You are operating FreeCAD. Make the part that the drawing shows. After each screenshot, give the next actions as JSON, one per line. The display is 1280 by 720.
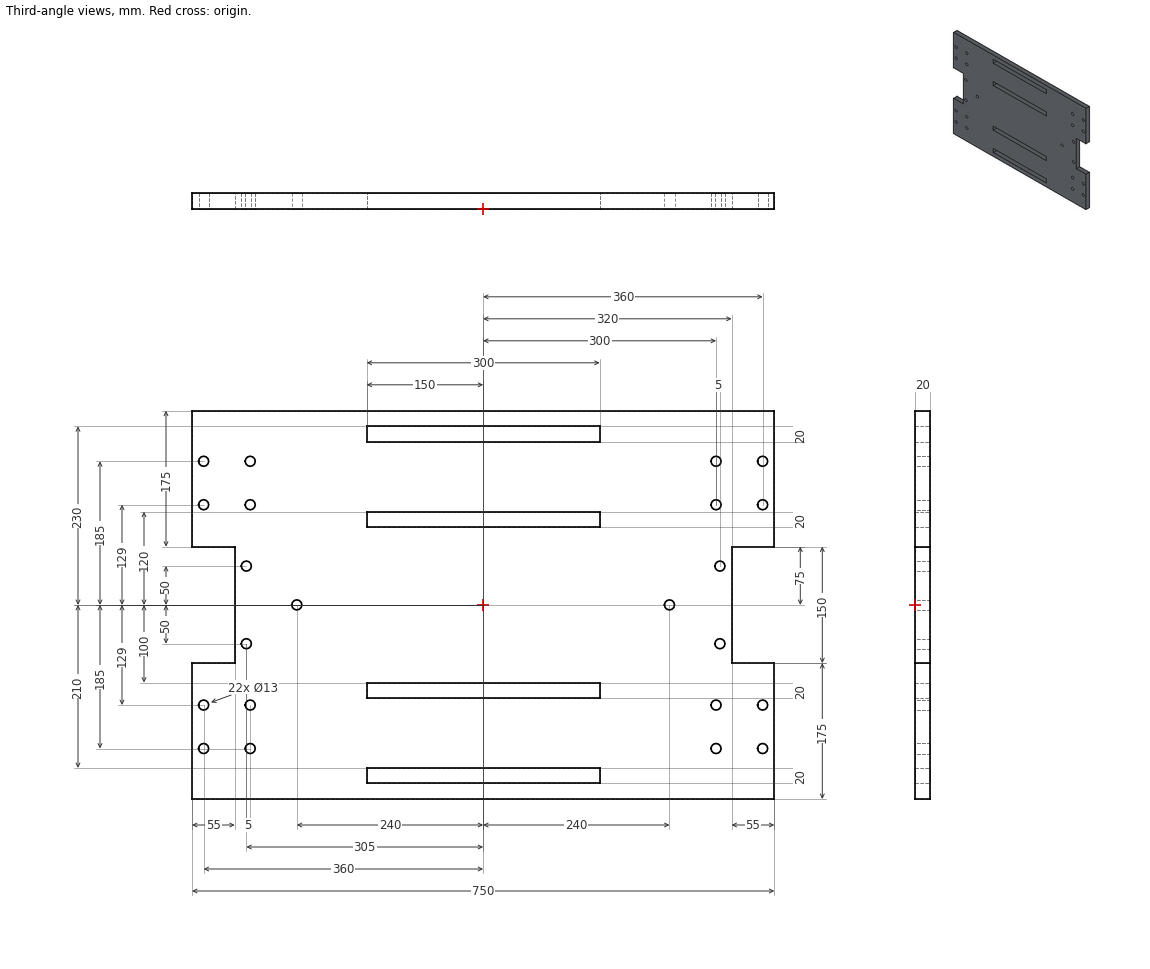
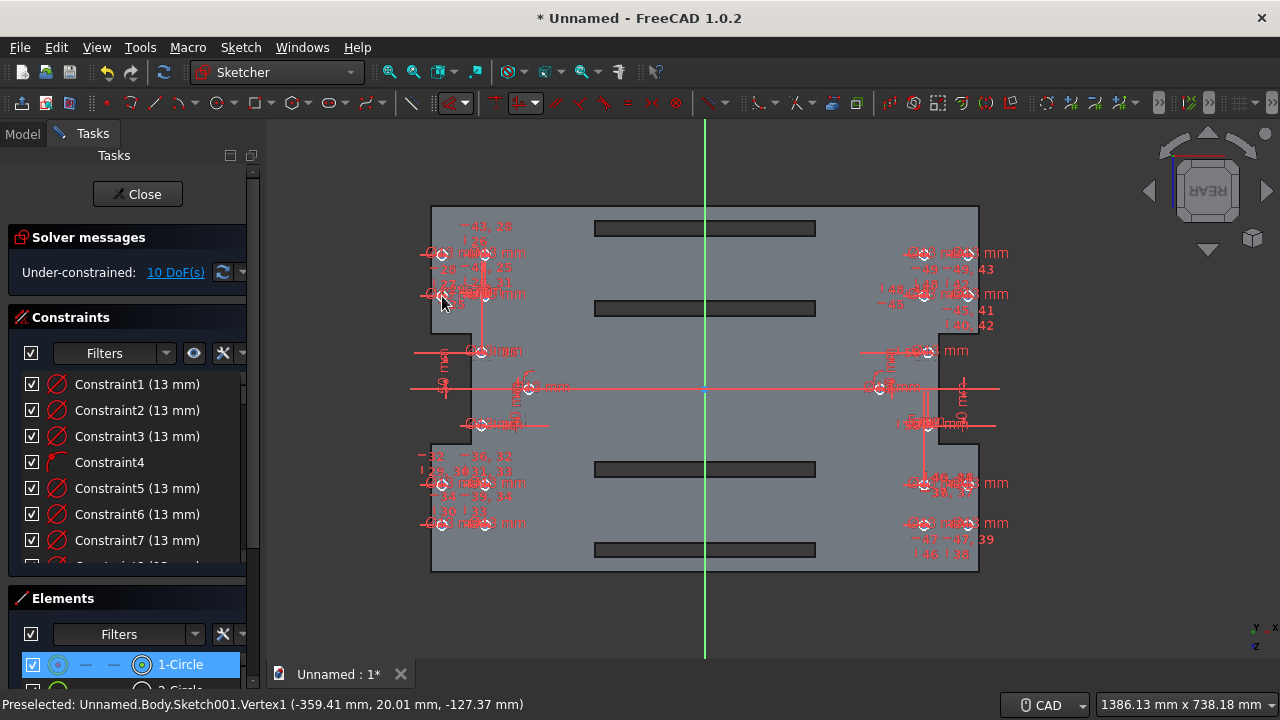
{"action": "key", "text": "l"}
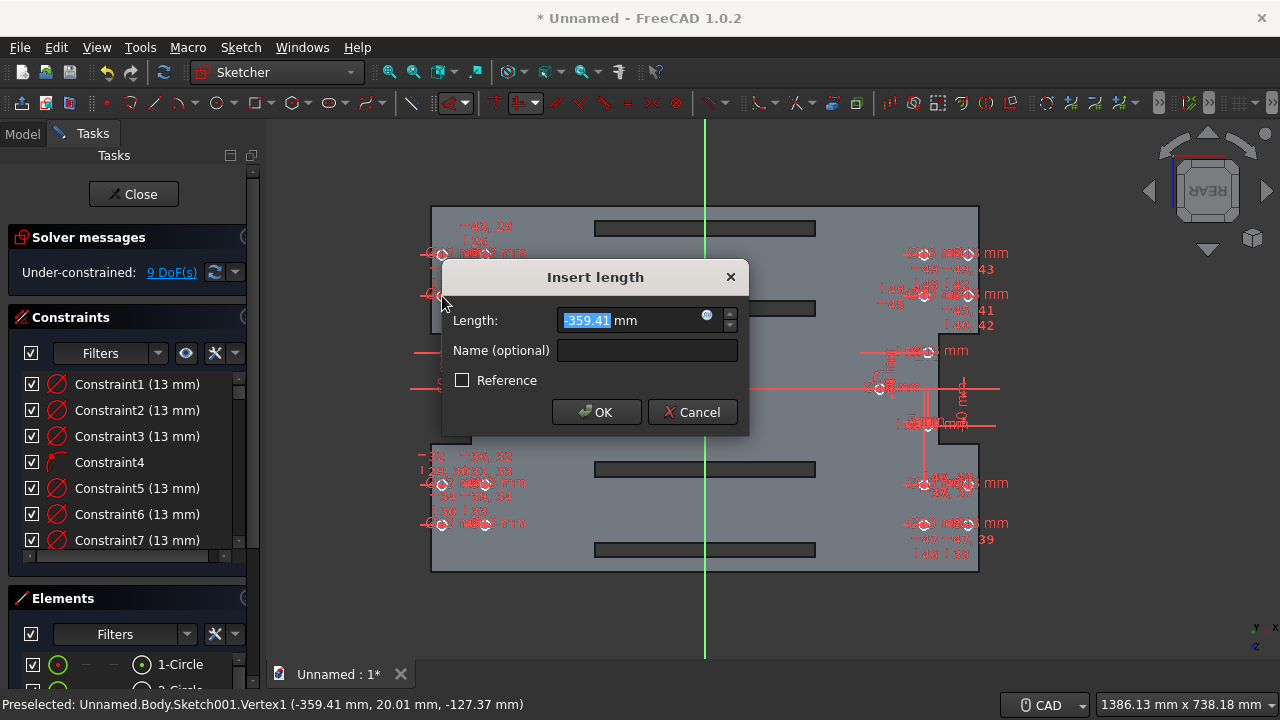
{"action": "type", "text": "-360"}
{"action": "key", "text": "Return"}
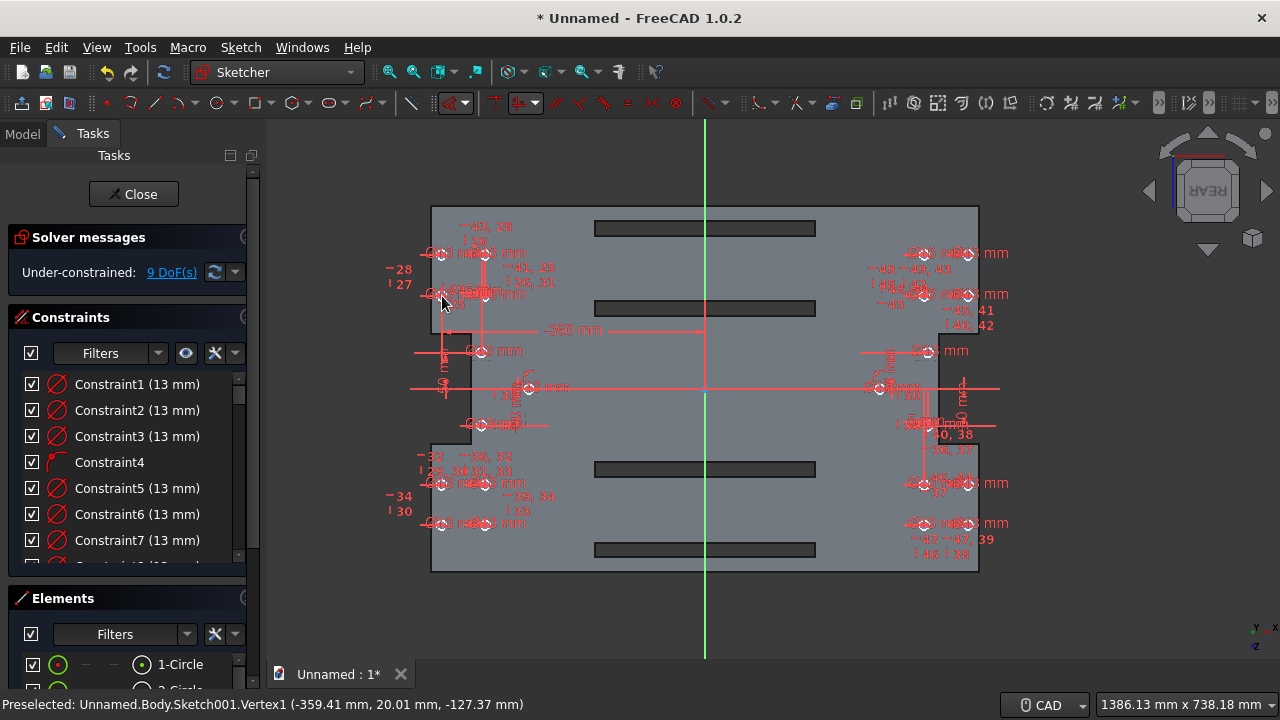
{"action": "left_click", "coordinate": [442, 296]}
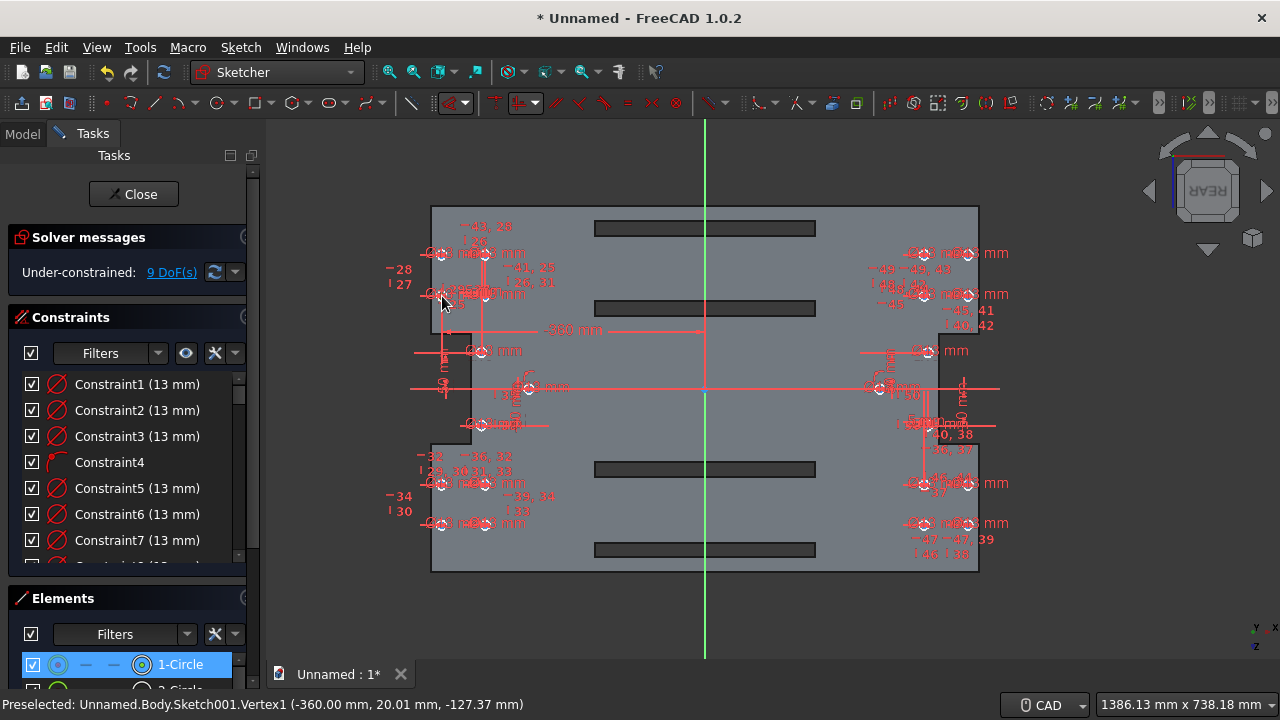
{"action": "key", "text": "i"}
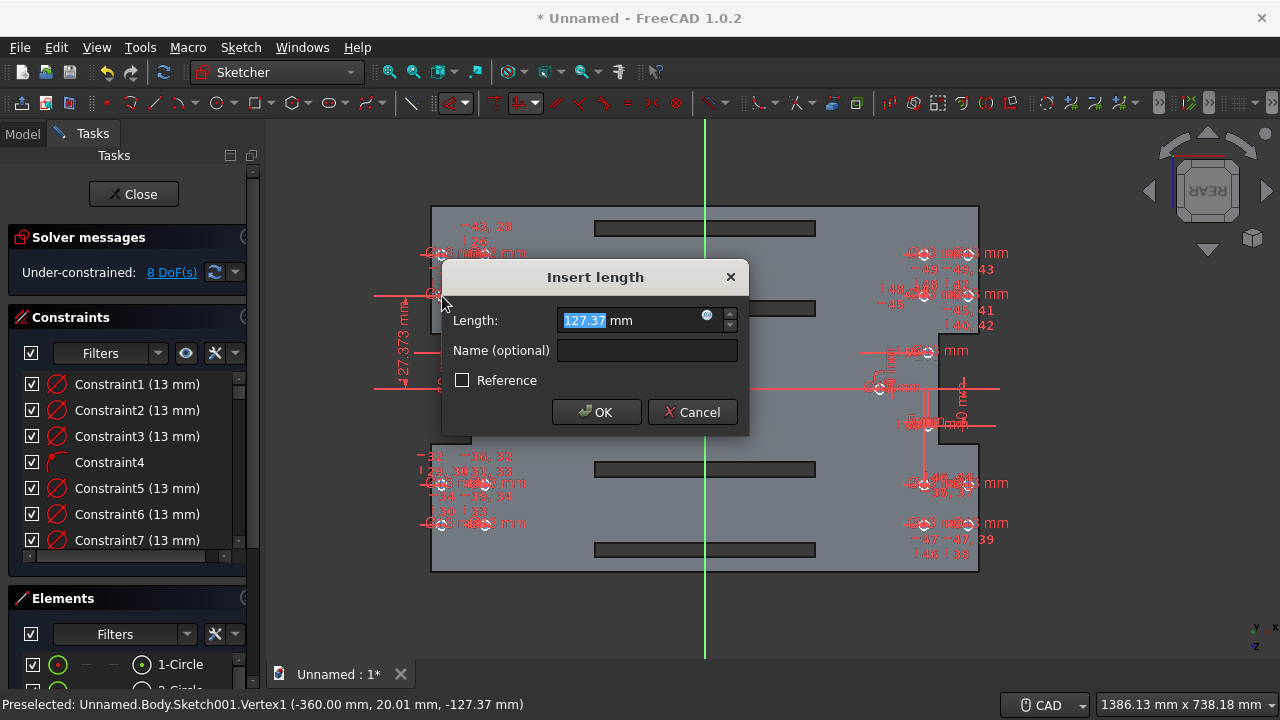
{"action": "type", "text": "129"}
{"action": "key", "text": "Return"}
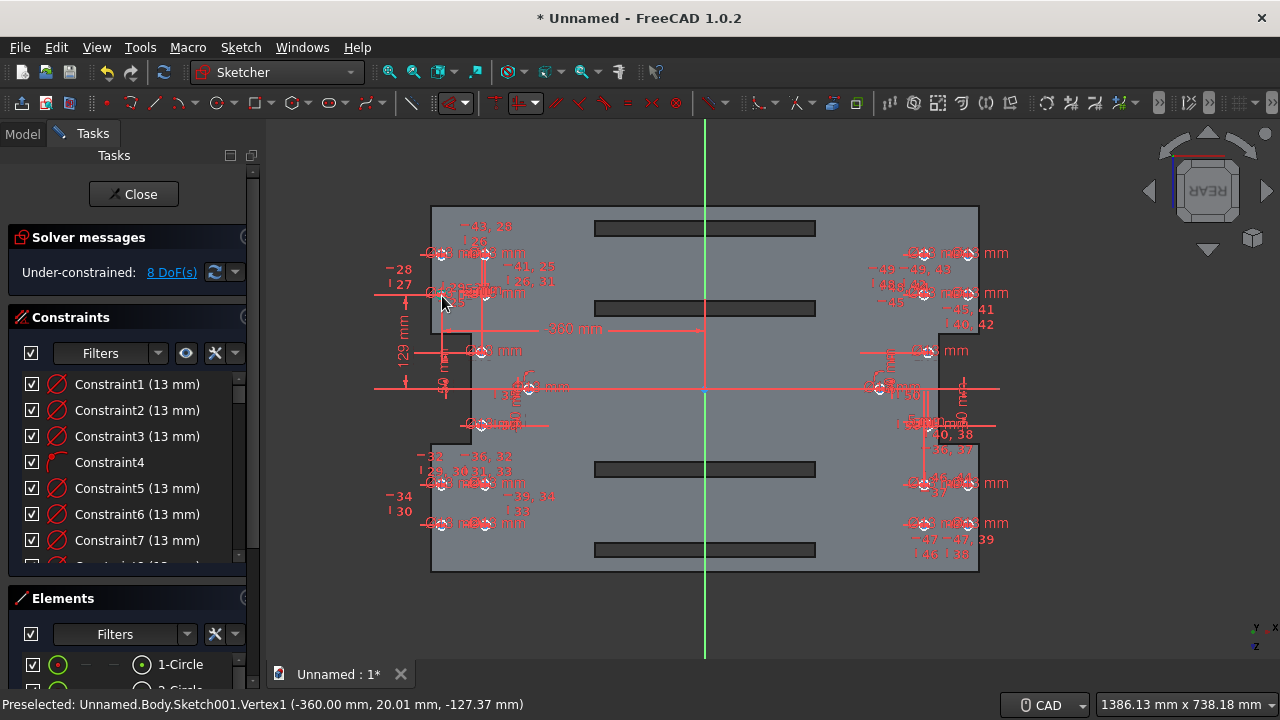
{"action": "left_click", "coordinate": [482, 353]}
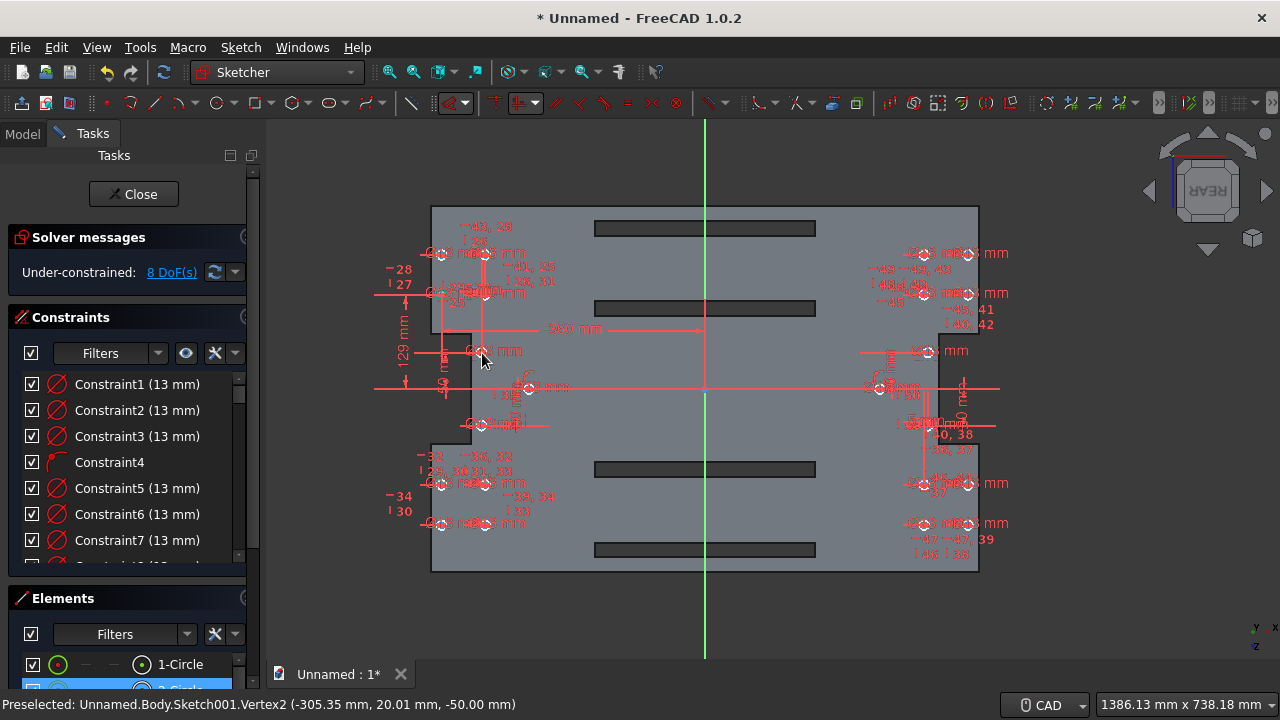
{"action": "left_click", "coordinate": [468, 104]}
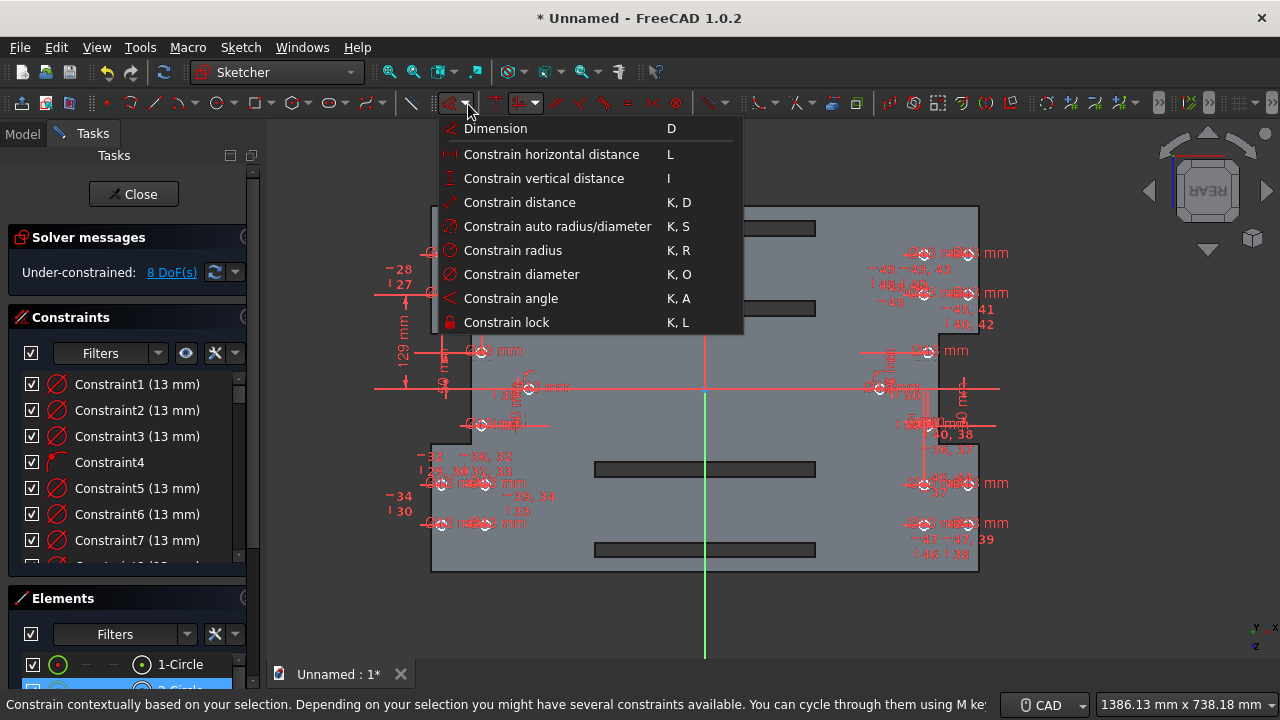
{"action": "left_click", "coordinate": [591, 154]}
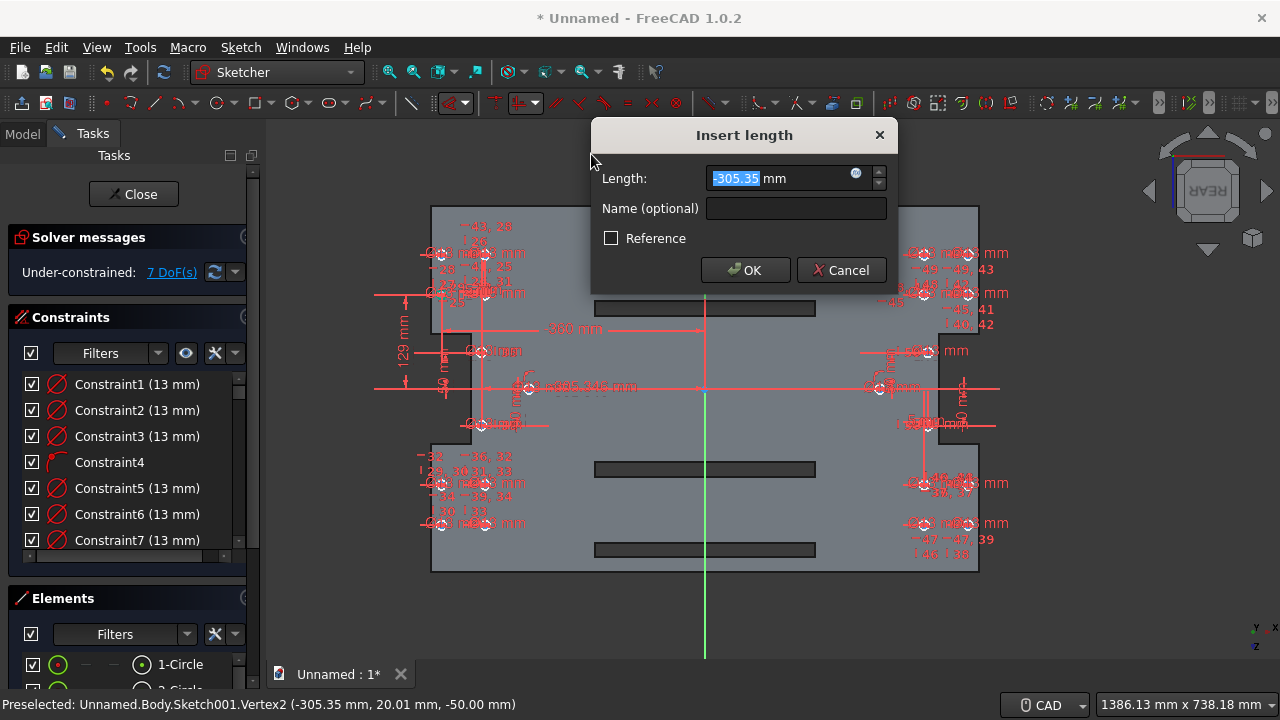
{"action": "type", "text": "-305"}
{"action": "key", "text": "Return"}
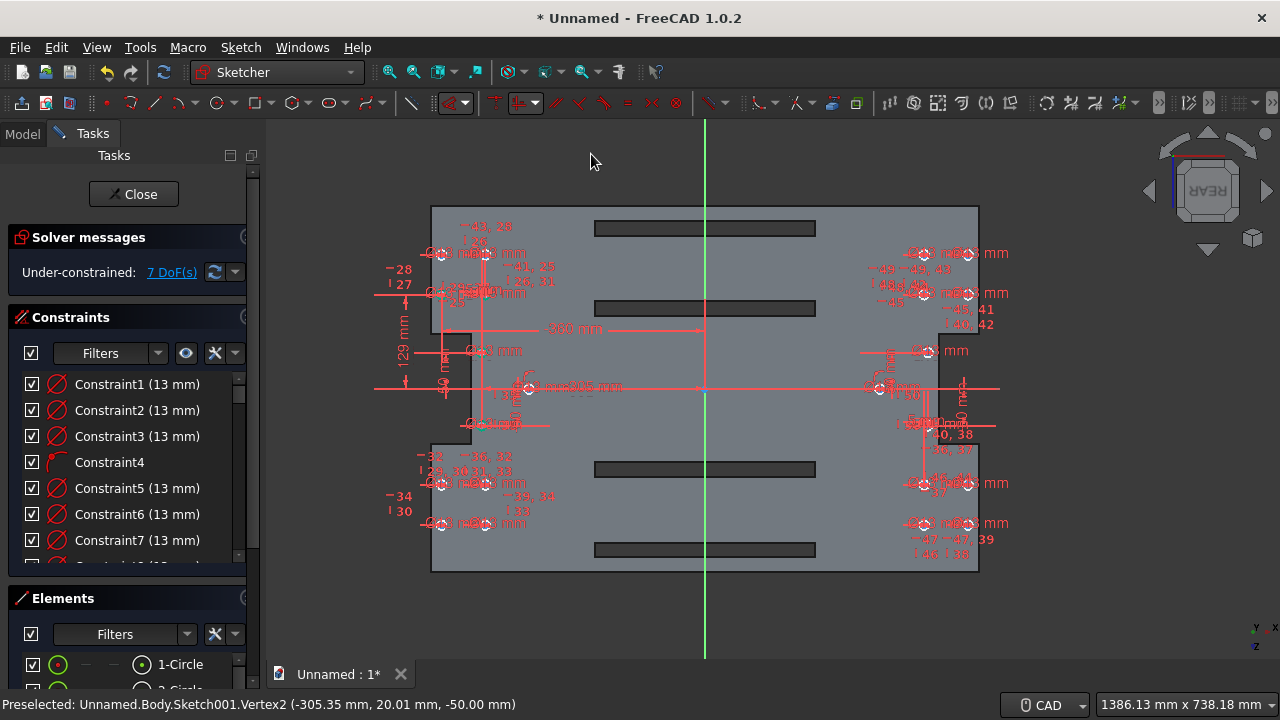
{"action": "left_click", "coordinate": [529, 389]}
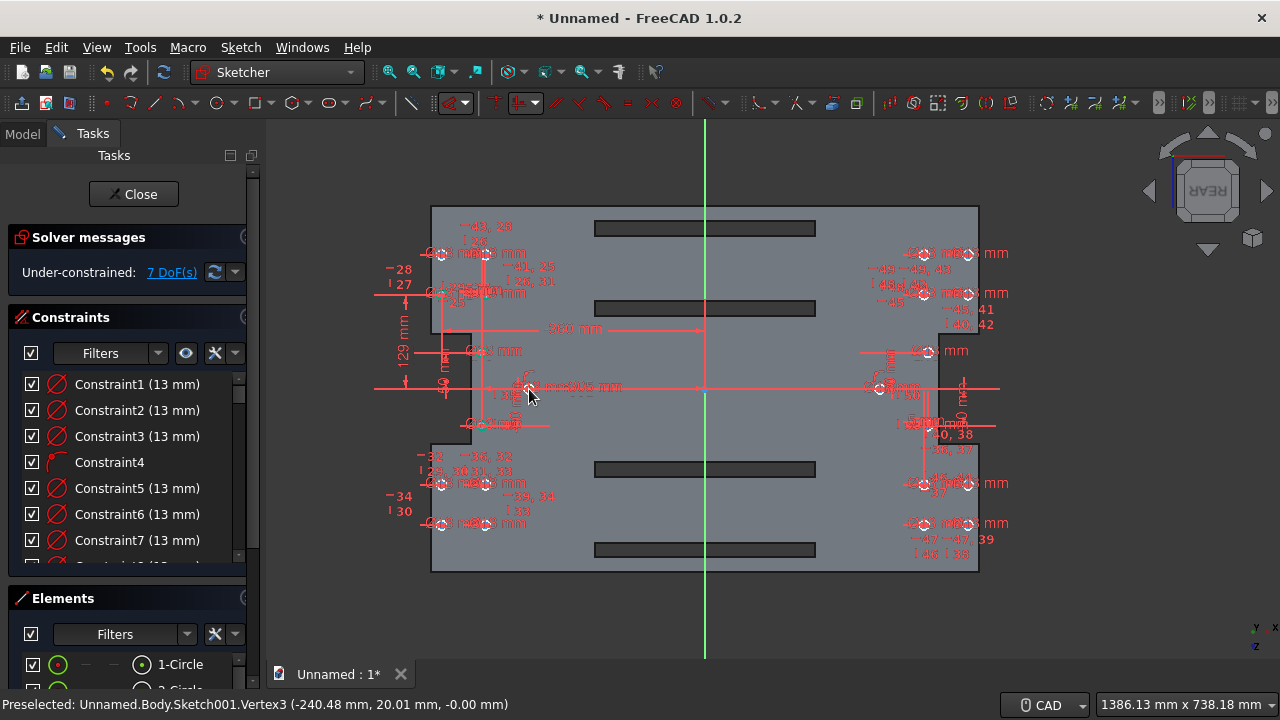
{"action": "key", "text": "l"}